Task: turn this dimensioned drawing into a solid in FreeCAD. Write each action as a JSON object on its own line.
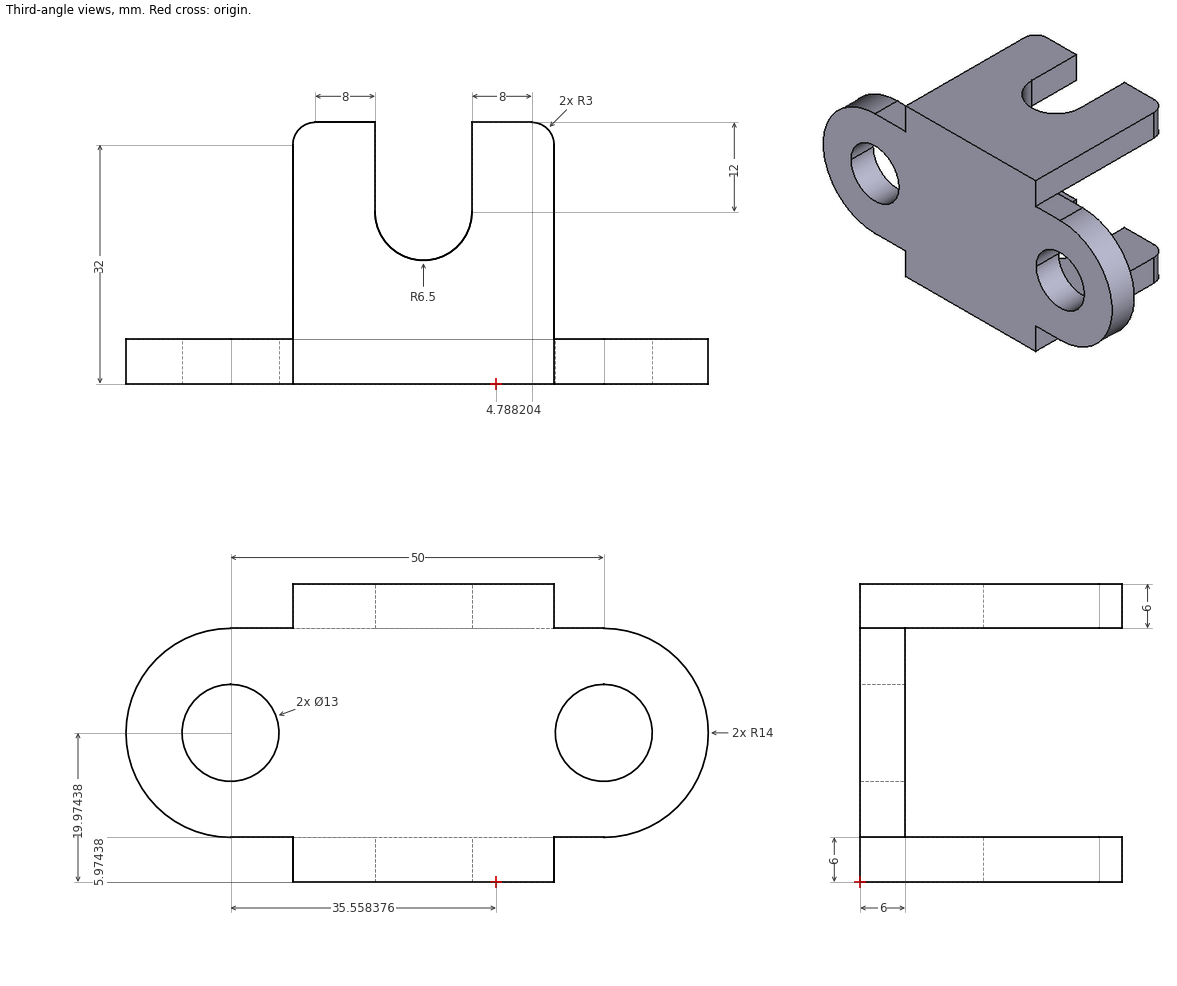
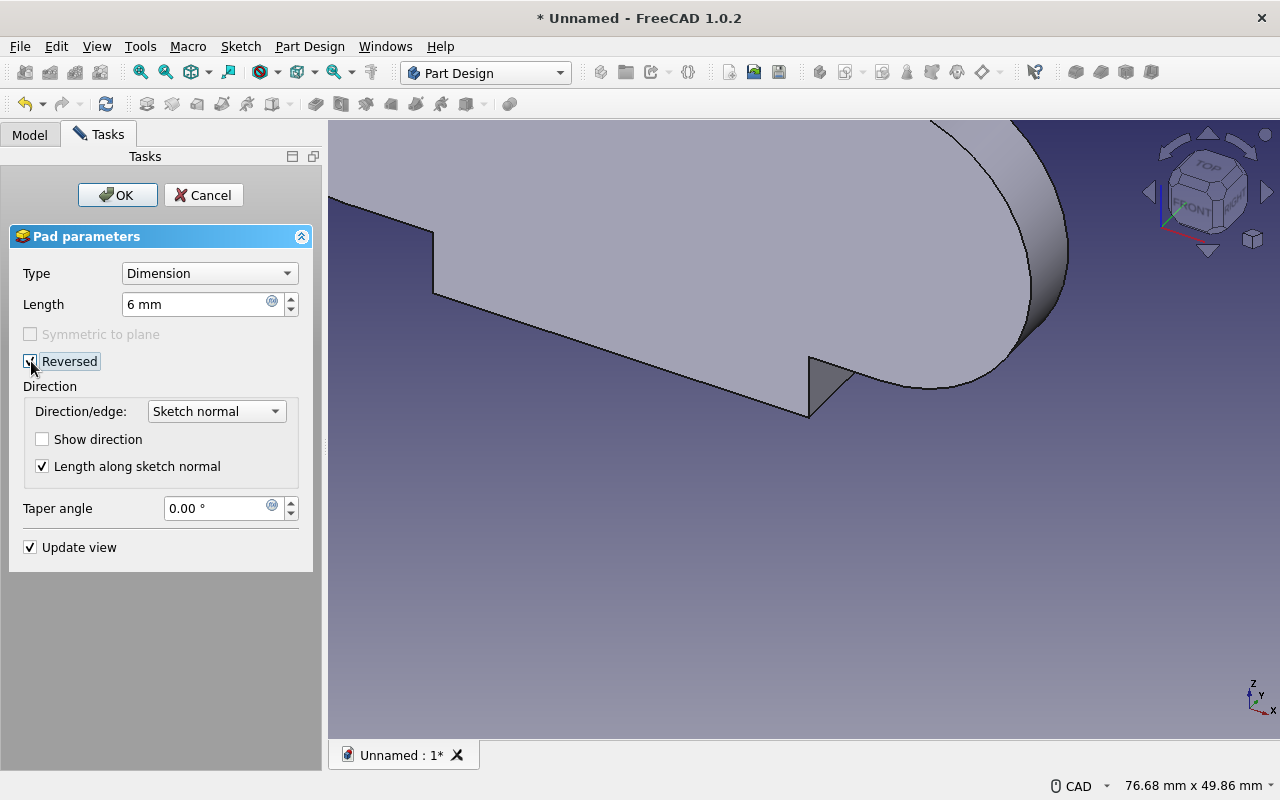
{"action": "left_click", "coordinate": [118, 195]}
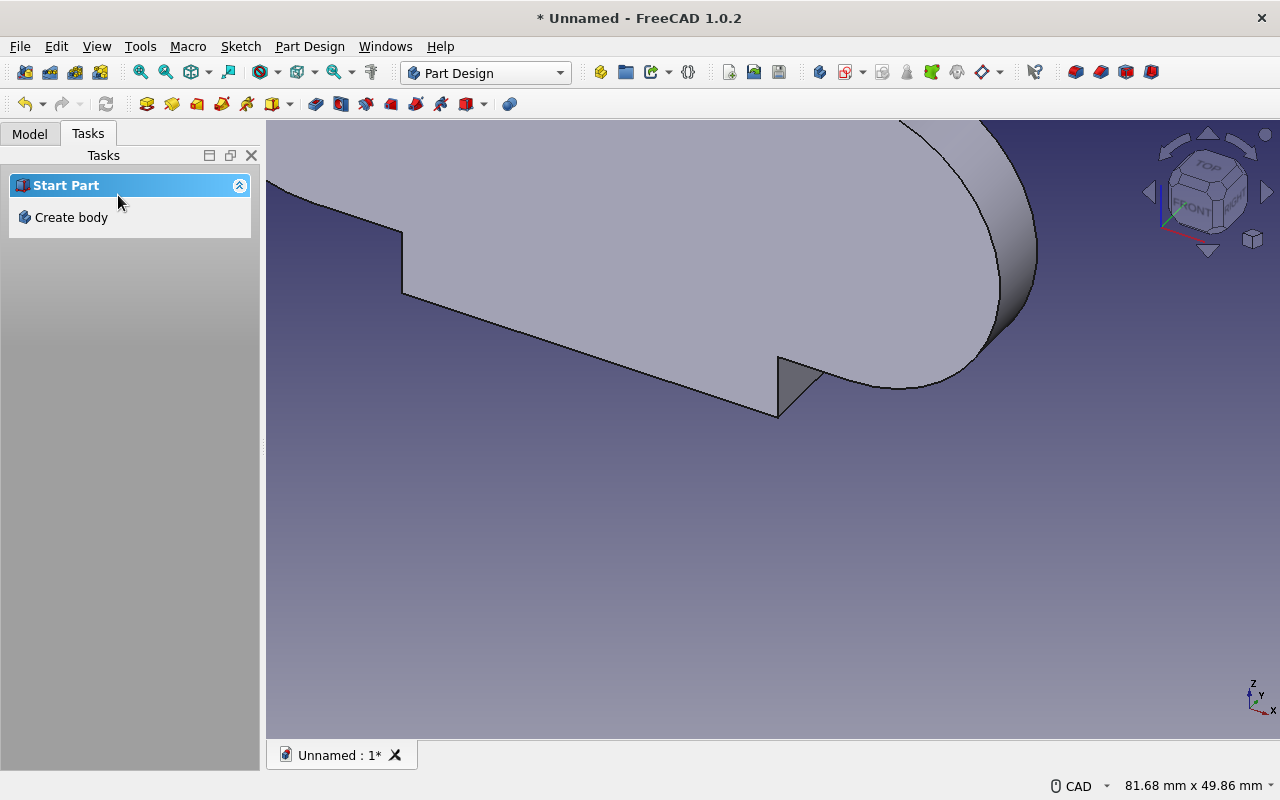
{"action": "left_click", "coordinate": [141, 72]}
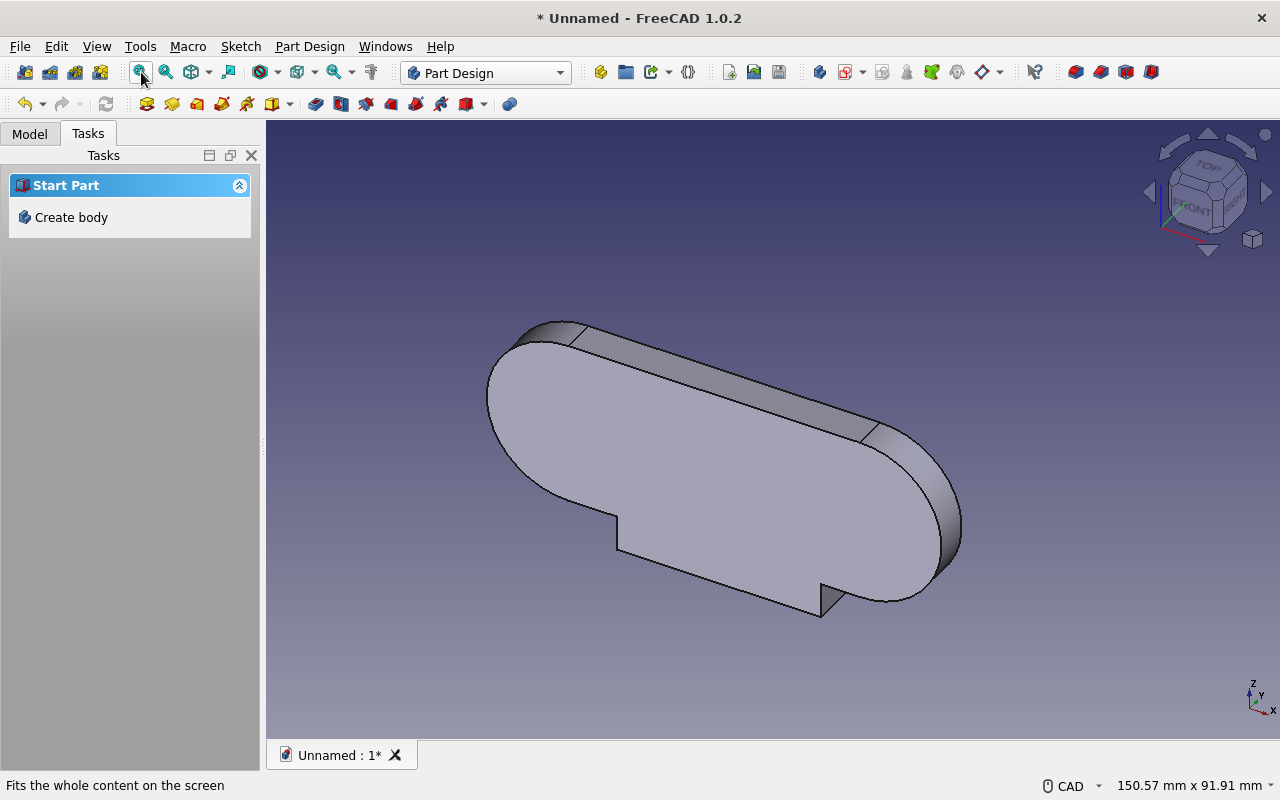
{"action": "key", "text": "4"}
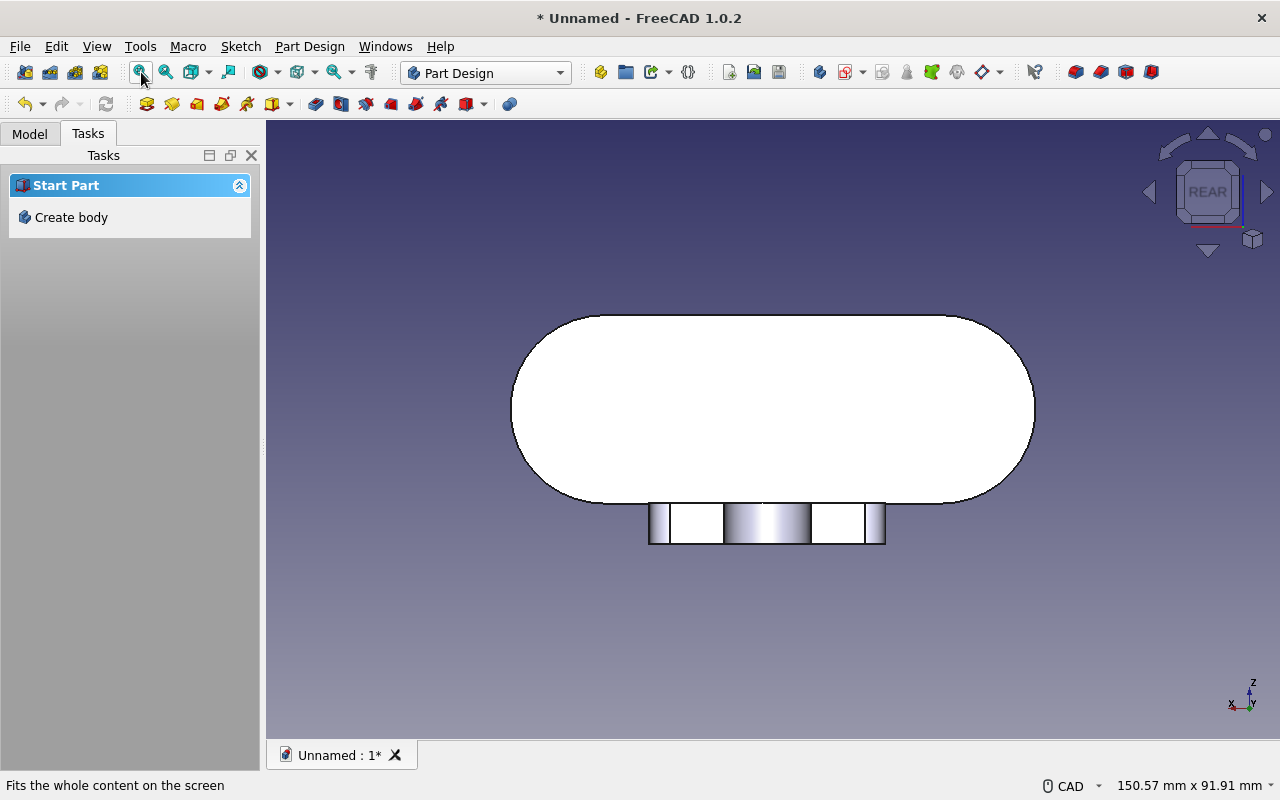
{"action": "left_click", "coordinate": [623, 408]}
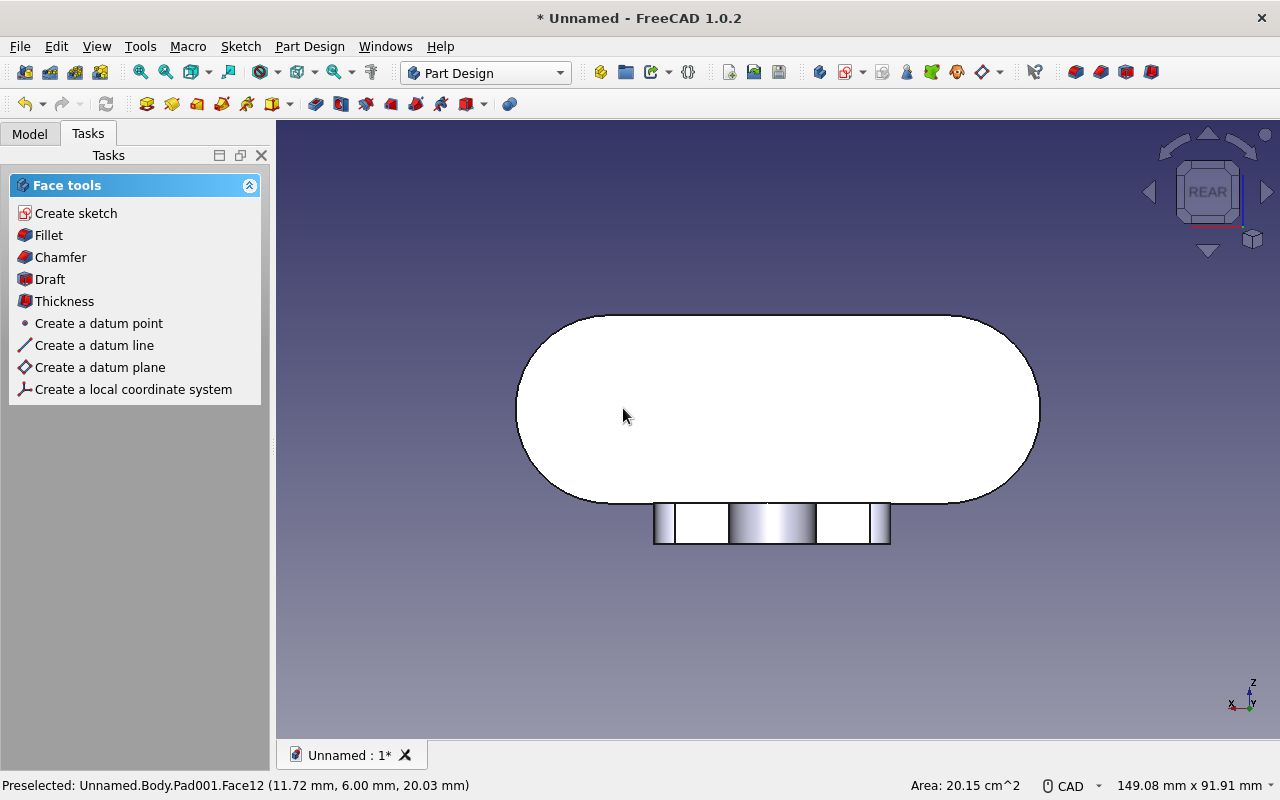
{"action": "left_click", "coordinate": [844, 72]}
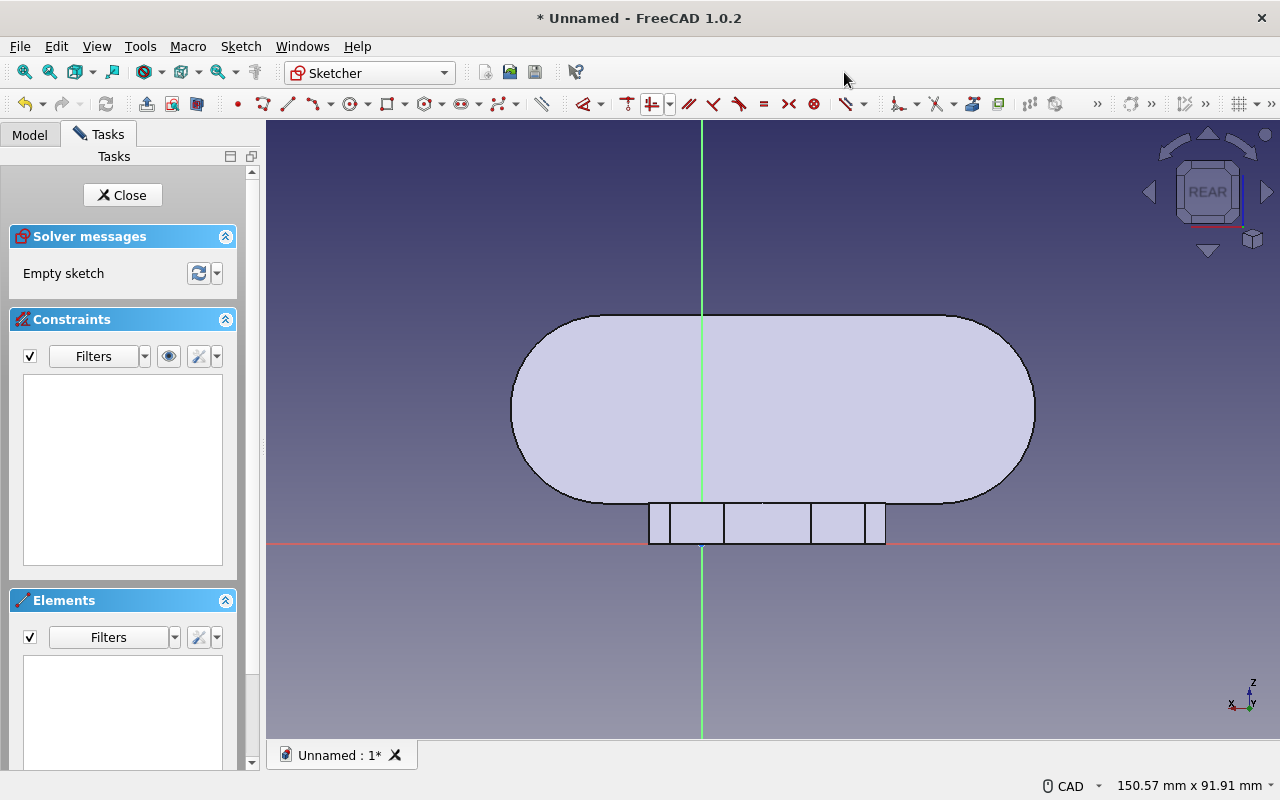
{"action": "left_click", "coordinate": [197, 104]}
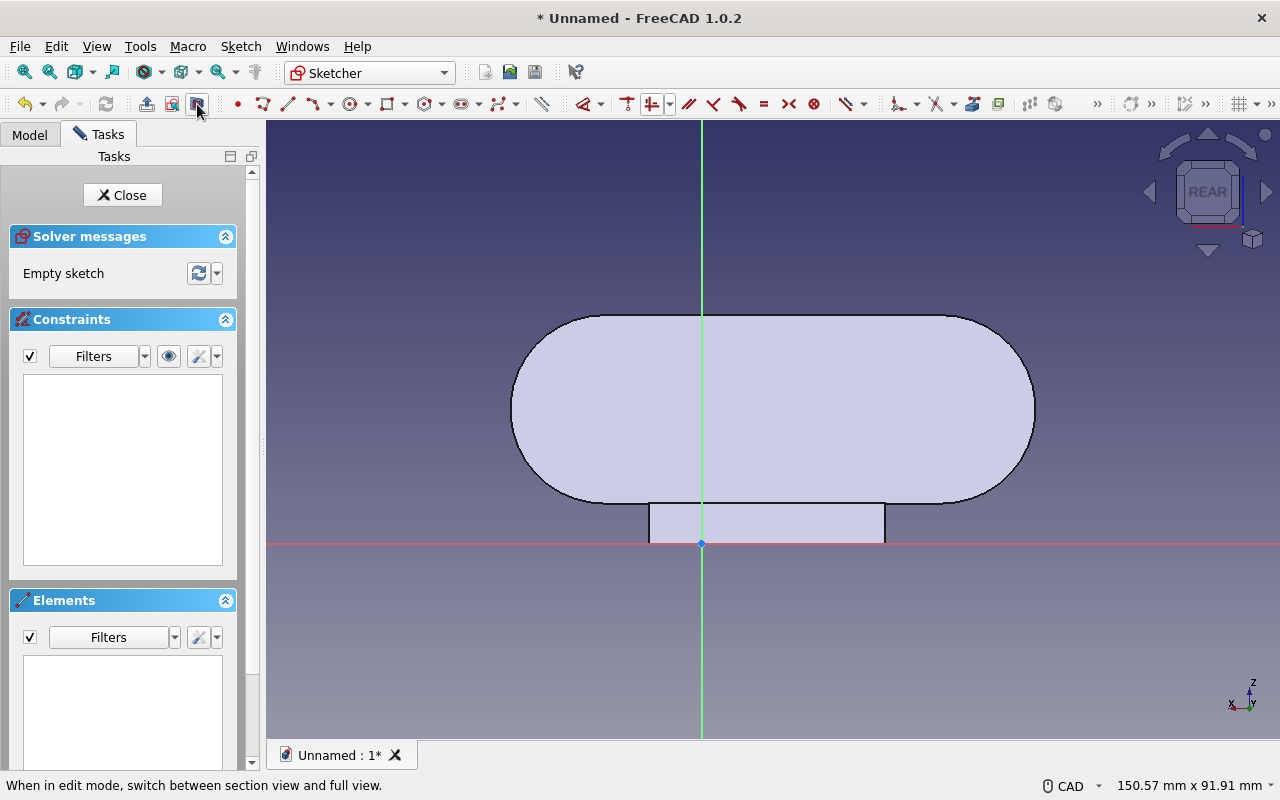
{"action": "scroll", "coordinate": [912, 506], "scroll_direction": "up", "scroll_amount": 2}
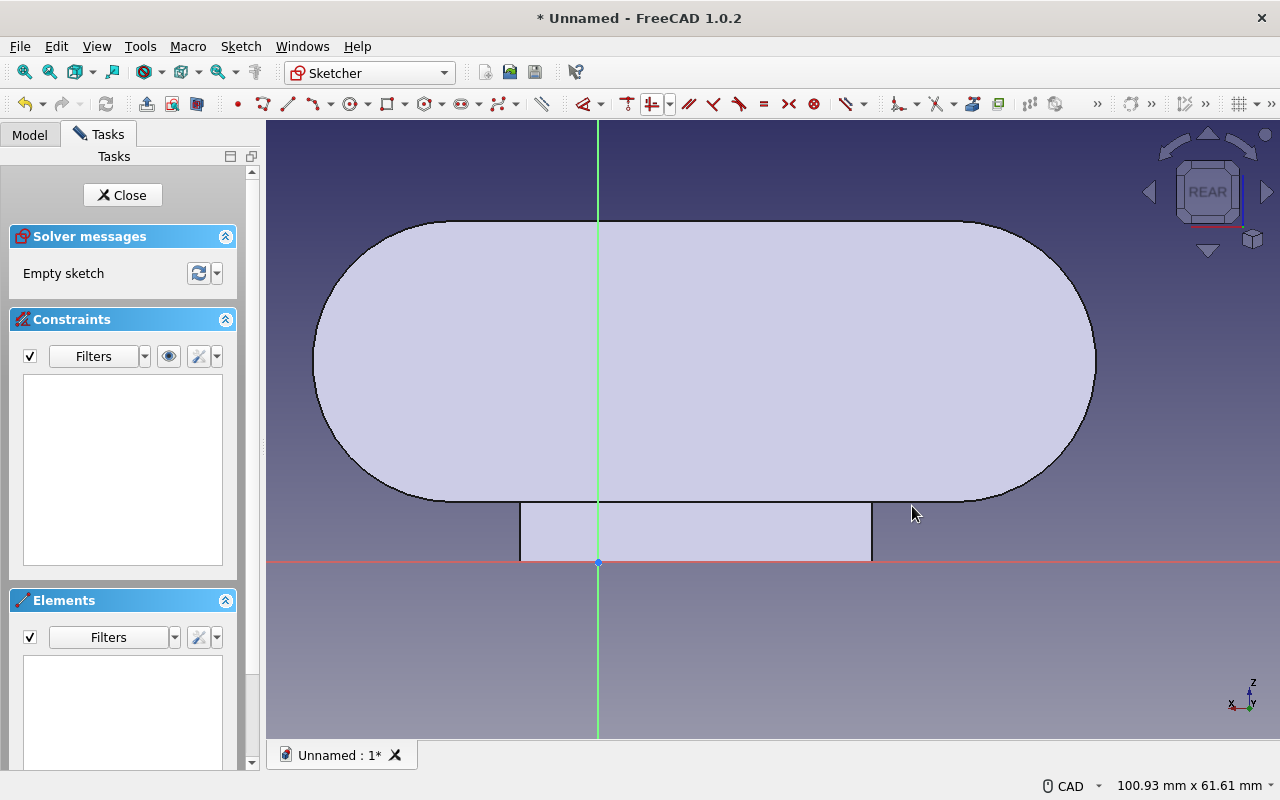
{"action": "left_click", "coordinate": [350, 104]}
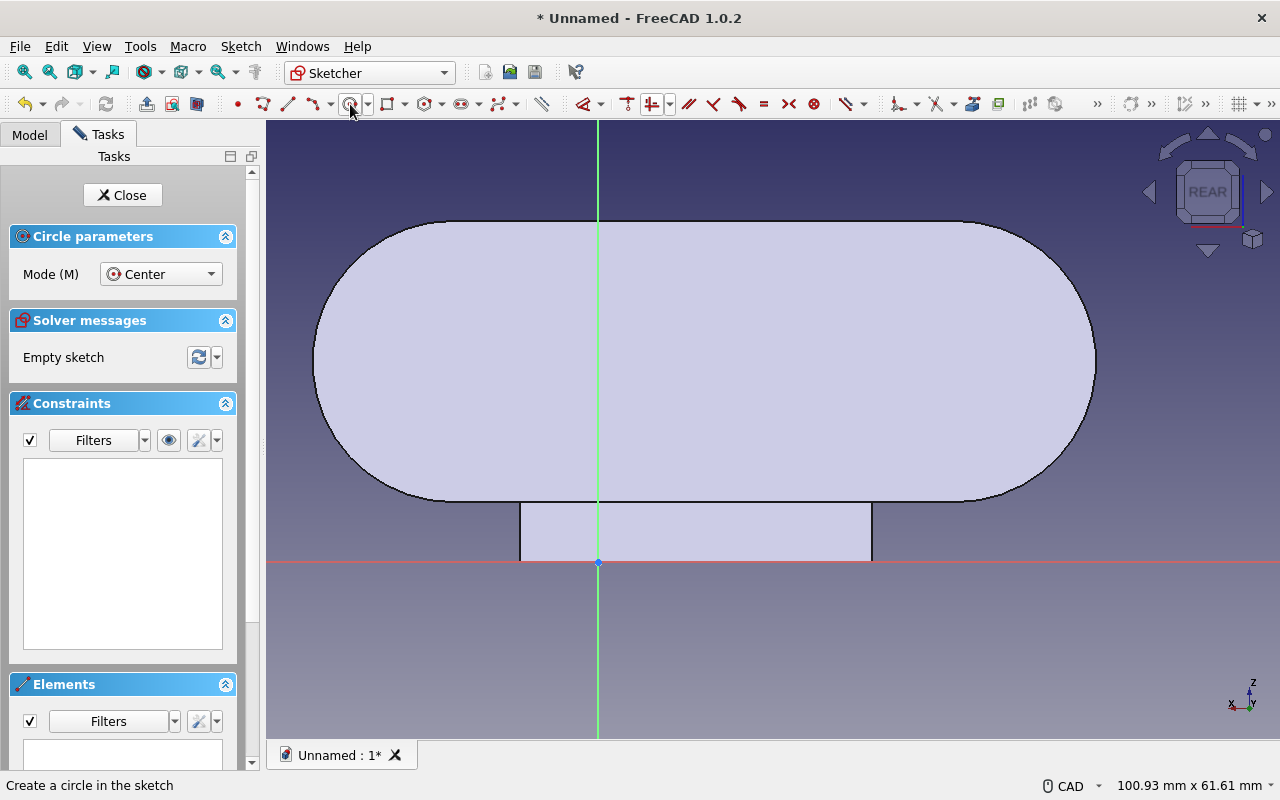
{"action": "left_click", "coordinate": [955, 362]}
{"action": "mouse_move", "coordinate": [1002, 315]}